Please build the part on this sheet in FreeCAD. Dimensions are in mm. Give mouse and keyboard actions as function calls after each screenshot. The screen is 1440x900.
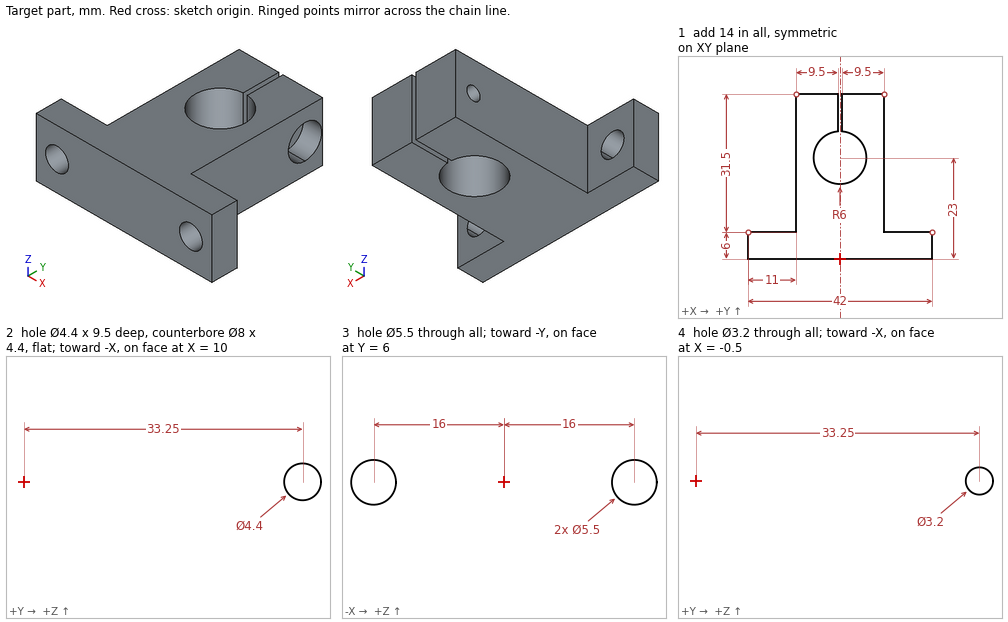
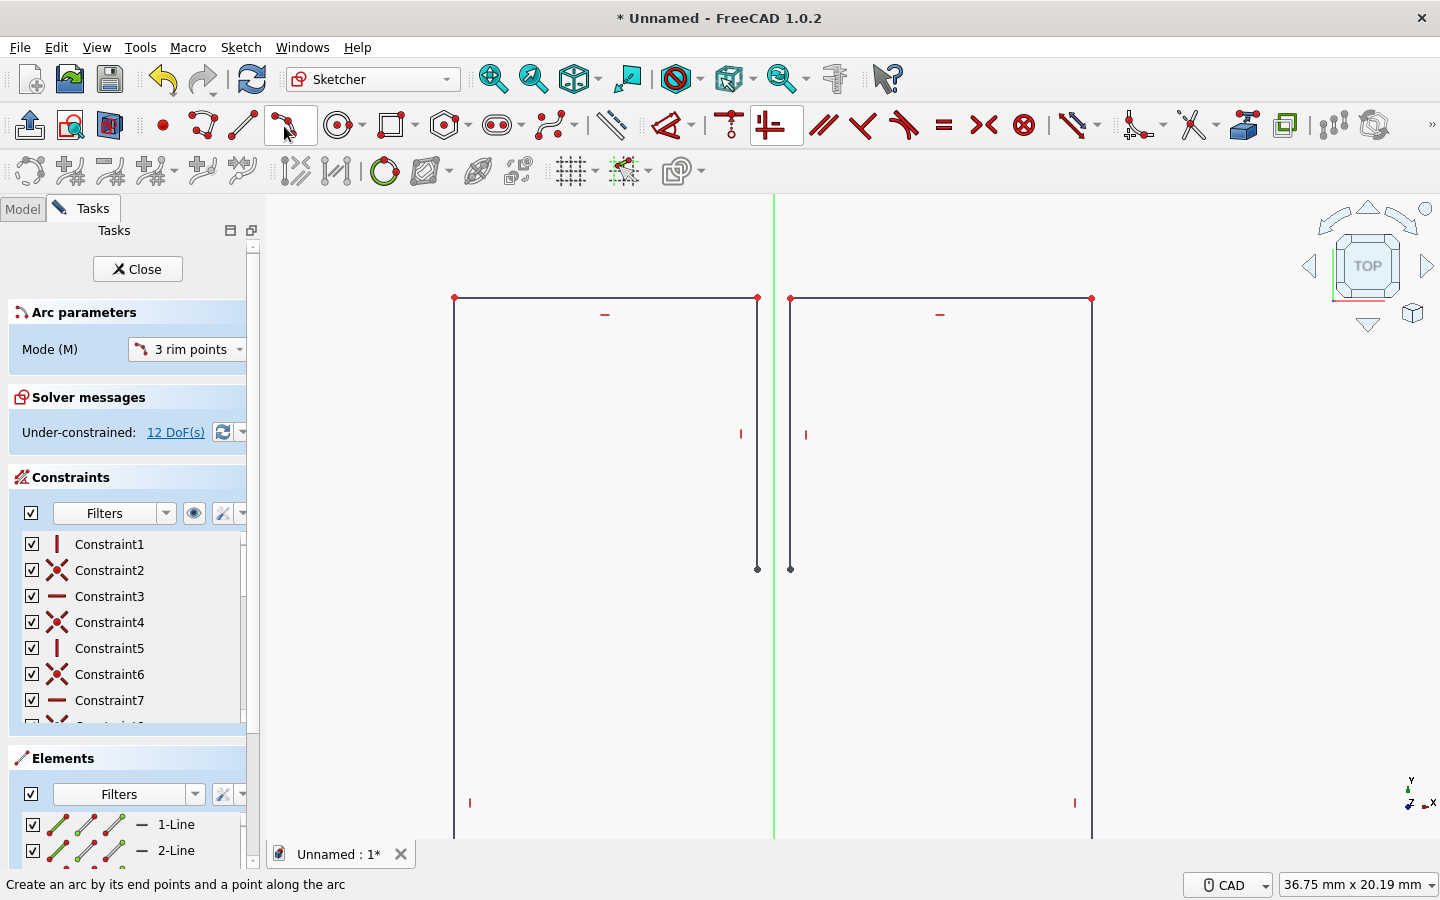
click(790, 570)
click(757, 570)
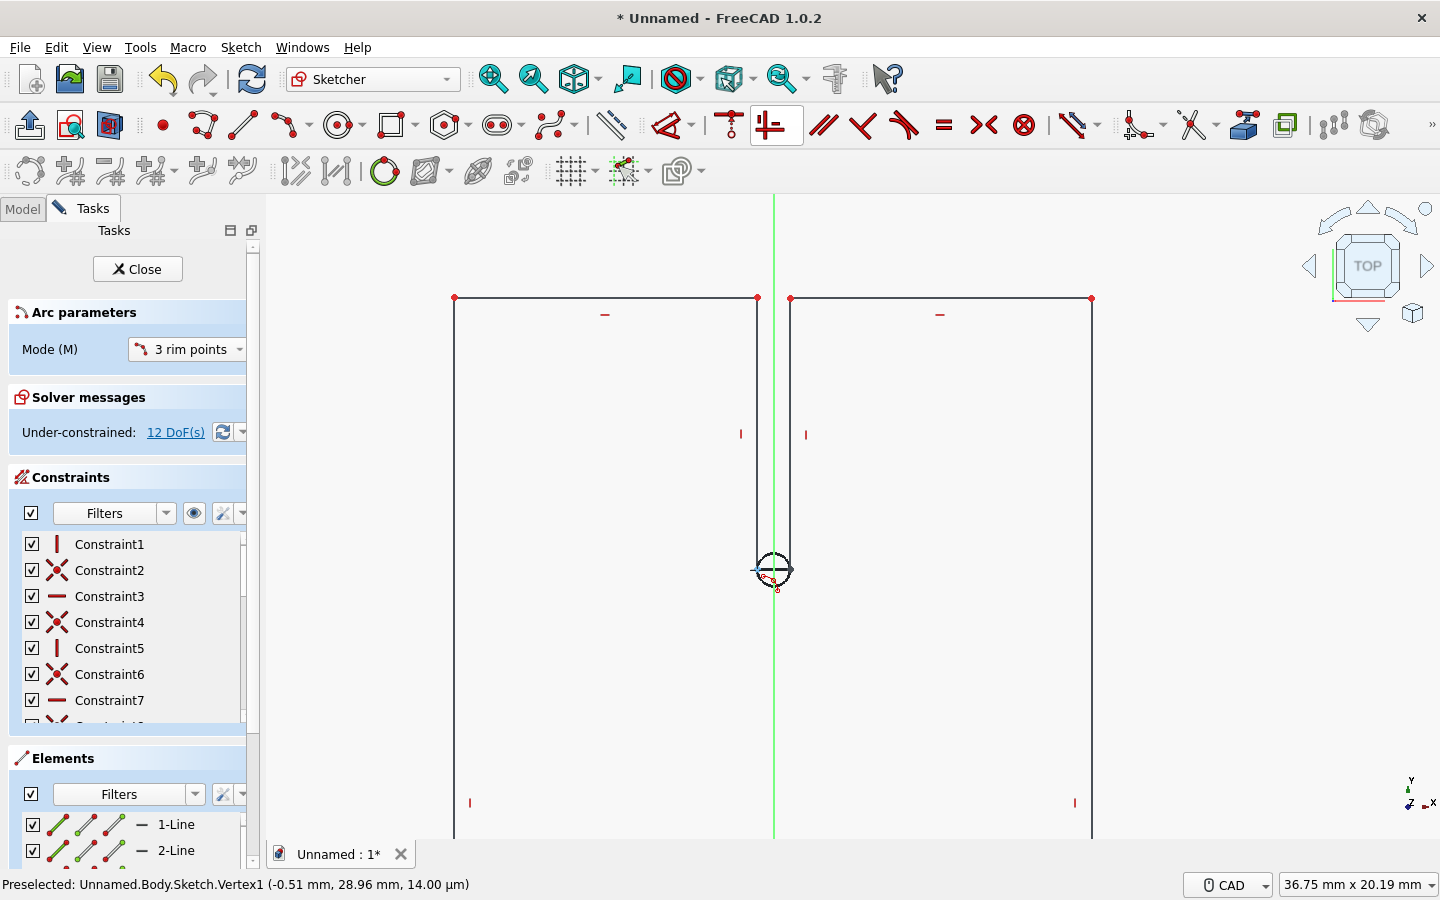
scroll(791, 296, down, 5)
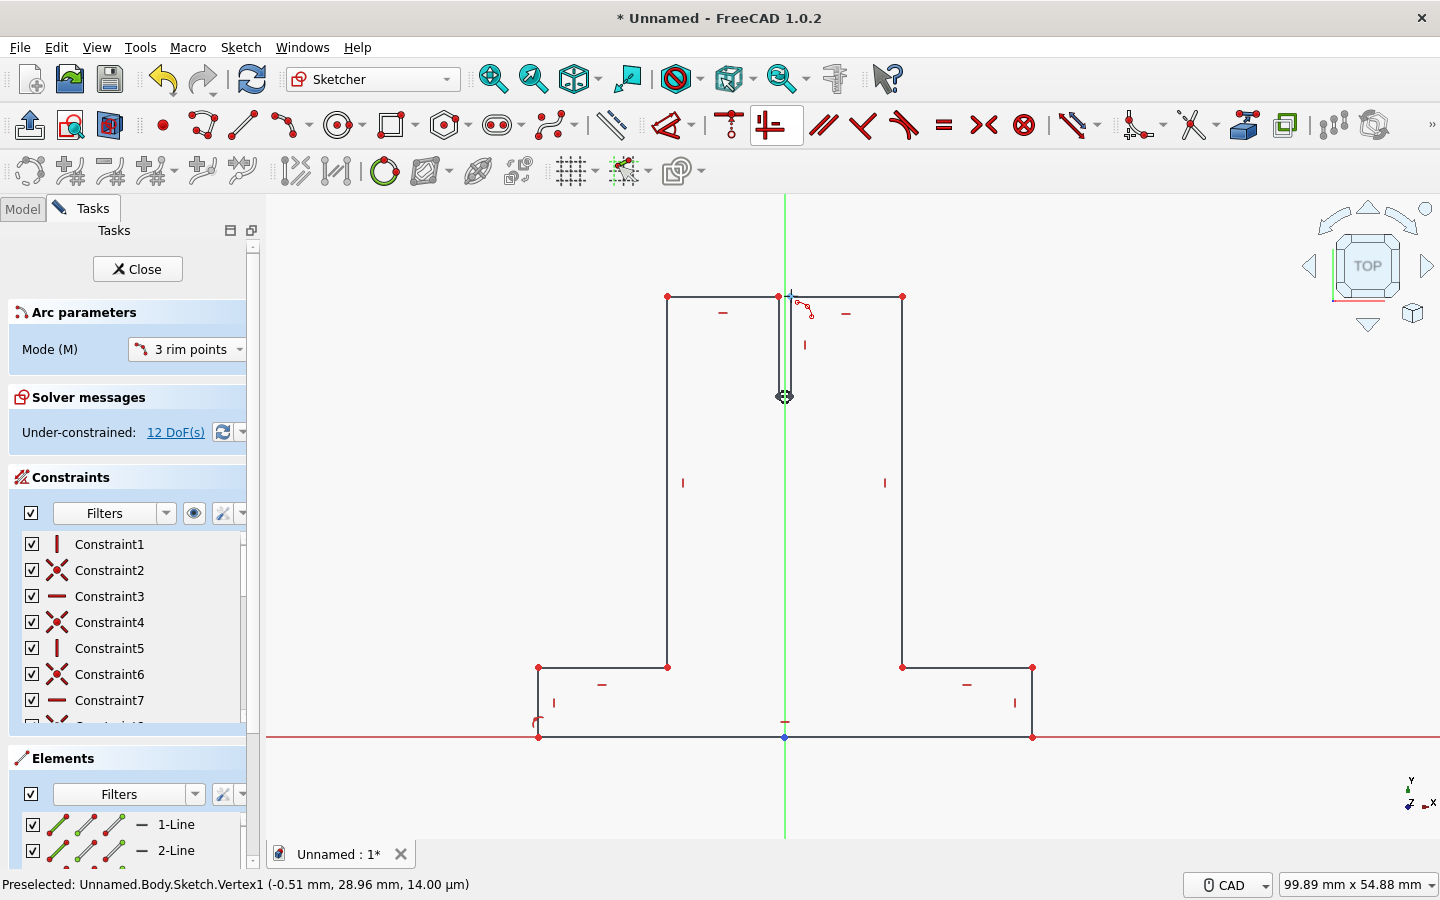
click(744, 525)
key(Escape)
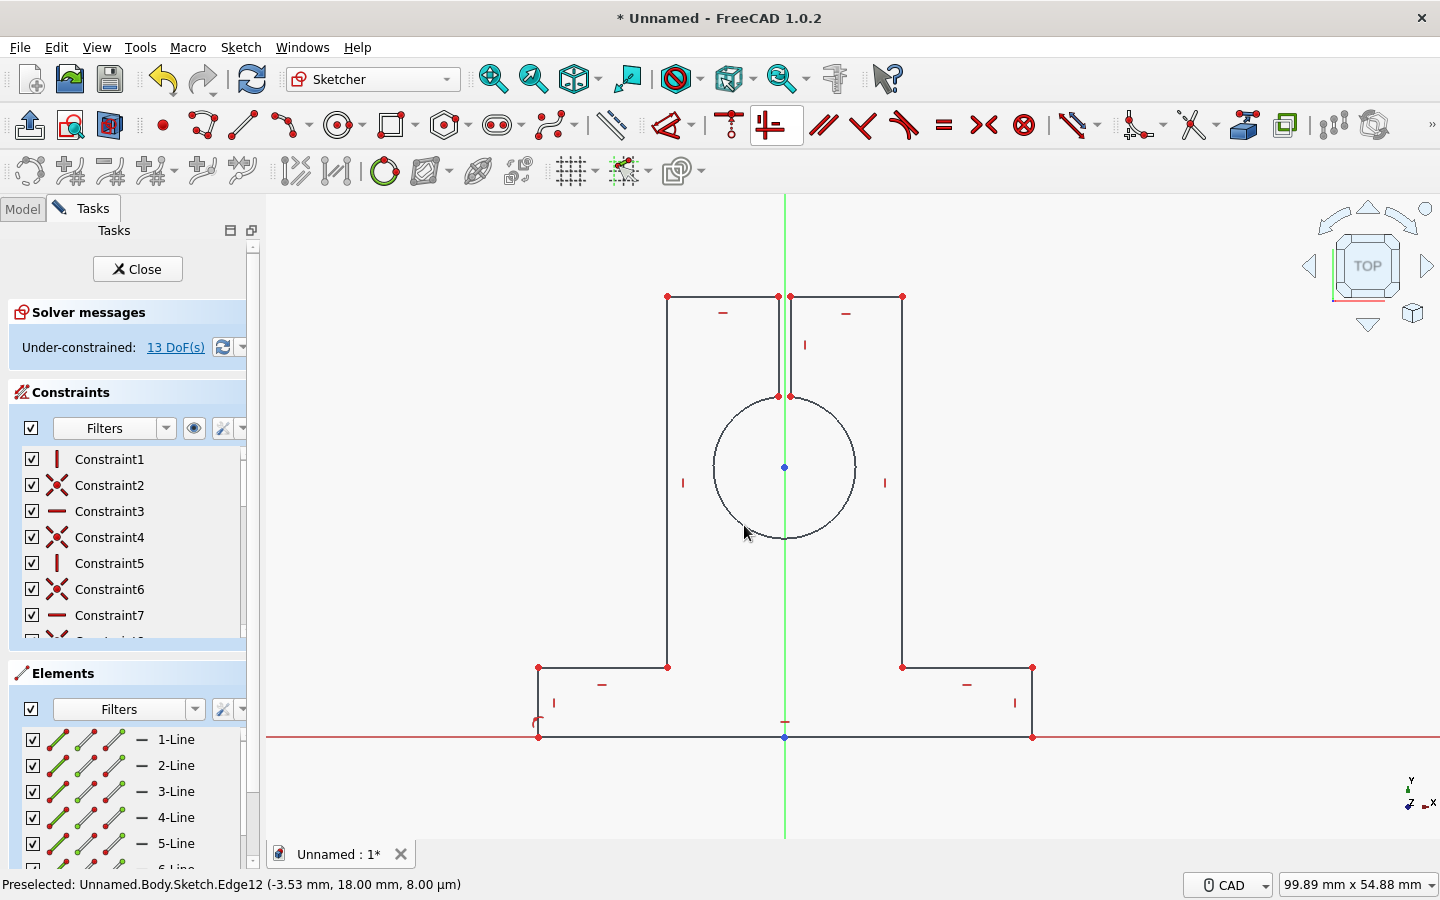
click(785, 468)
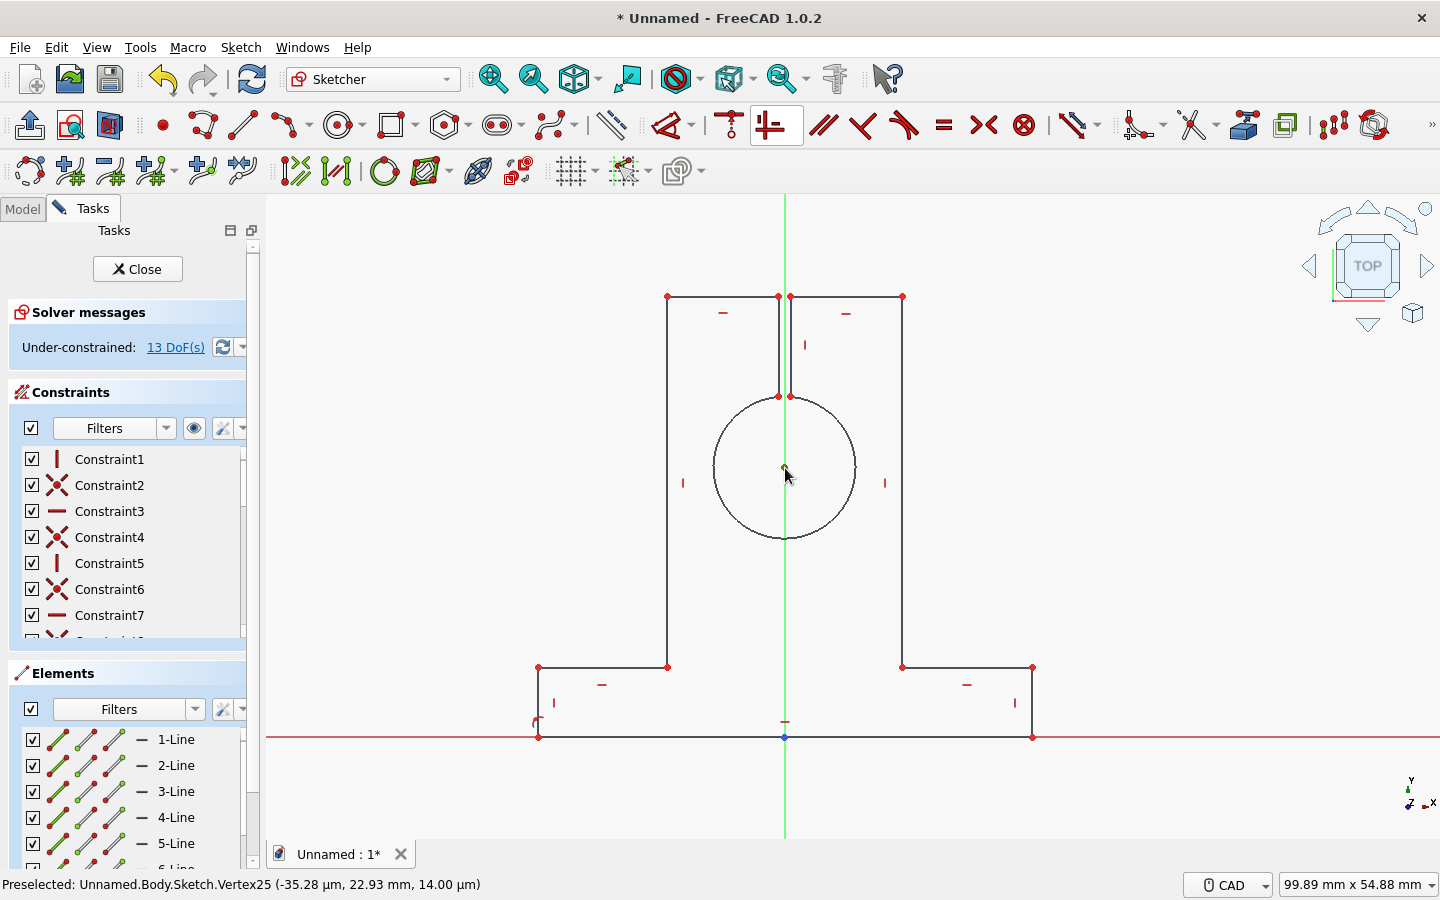
click(785, 769)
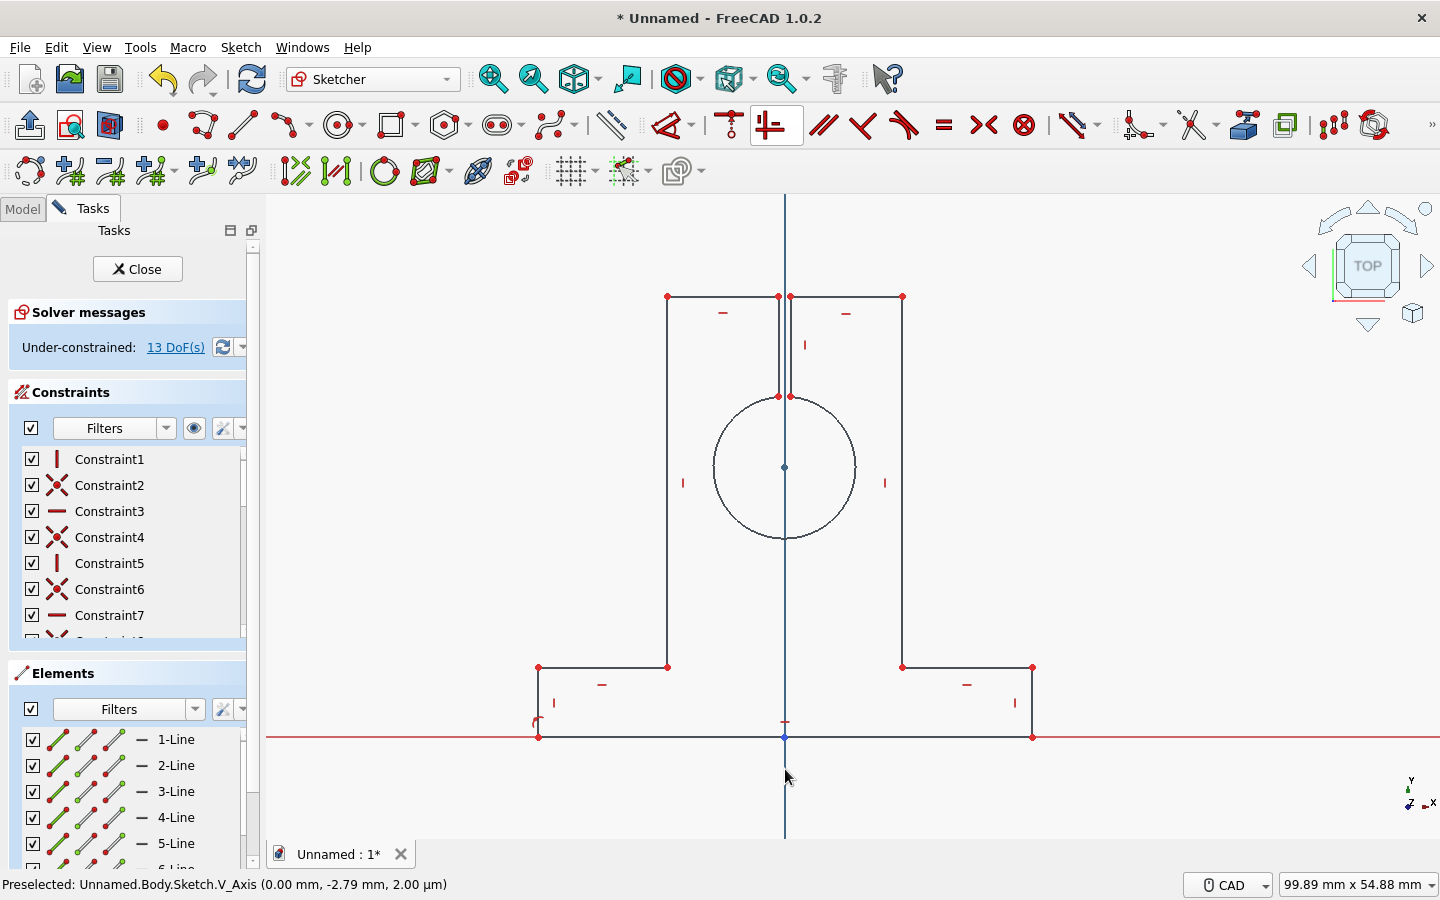
click(730, 126)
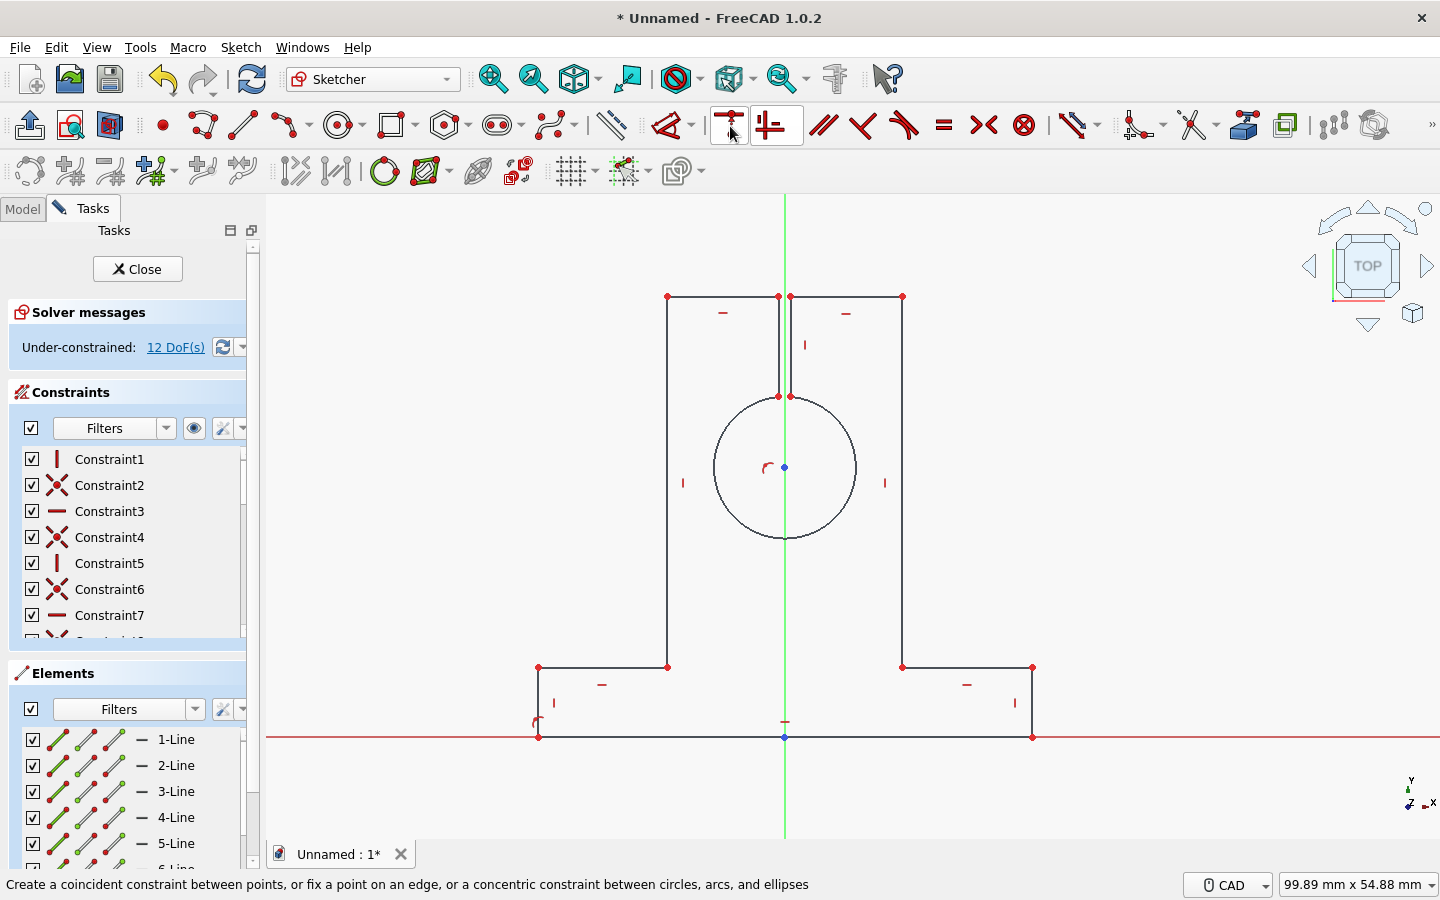
click(538, 668)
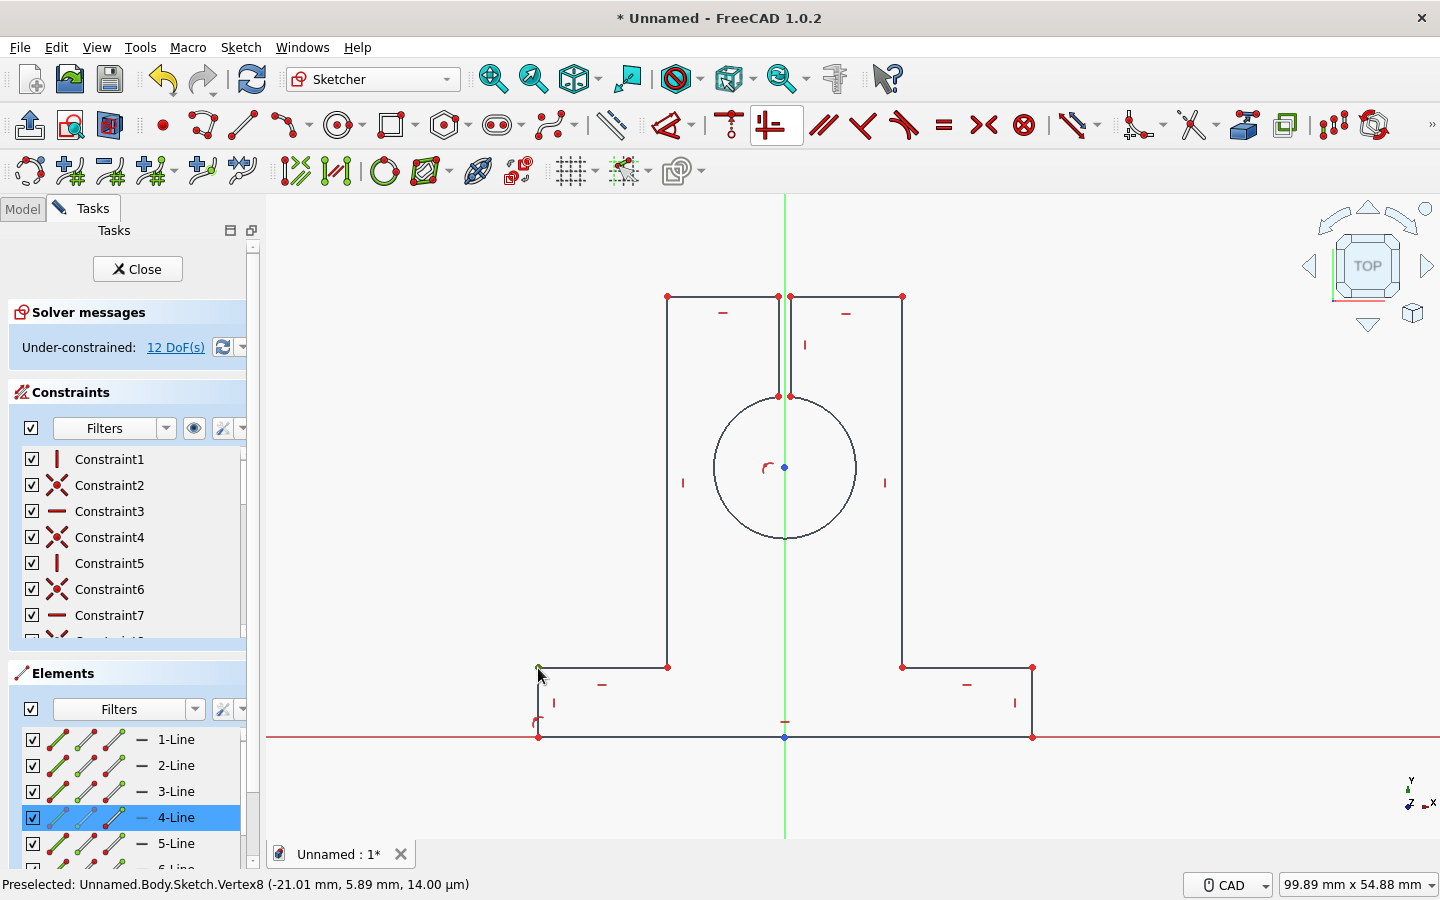
click(1032, 668)